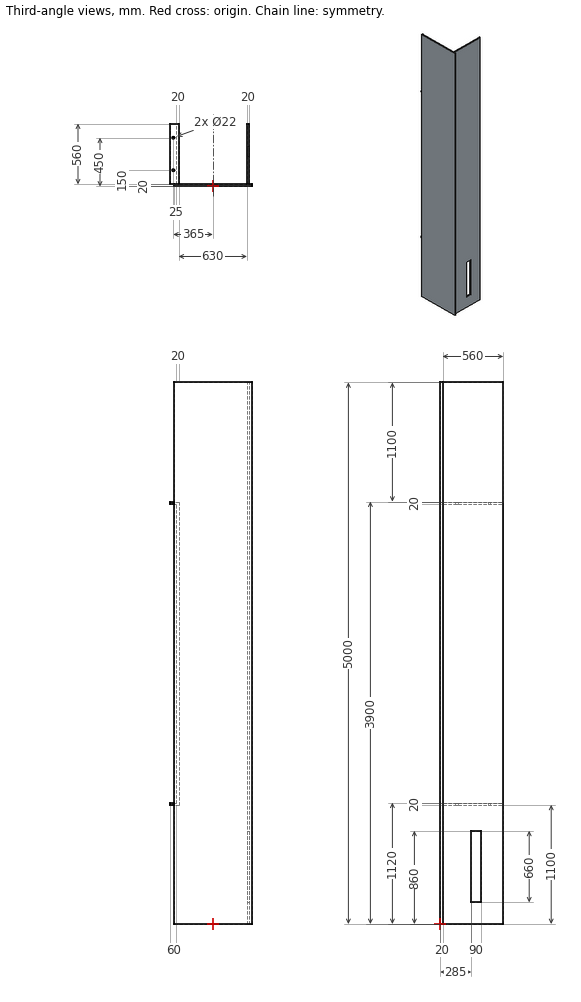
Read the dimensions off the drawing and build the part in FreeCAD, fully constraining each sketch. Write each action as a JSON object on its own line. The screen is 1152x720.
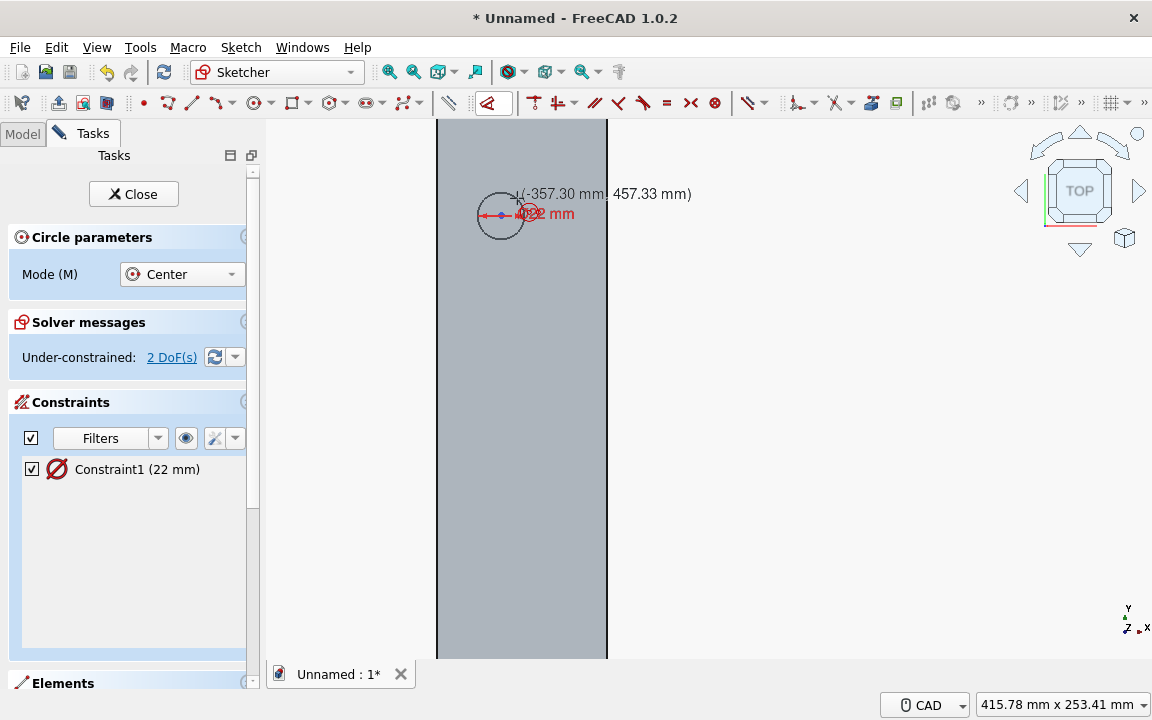
{"action": "scroll", "coordinate": [502, 218], "scroll_direction": "down", "scroll_amount": 5}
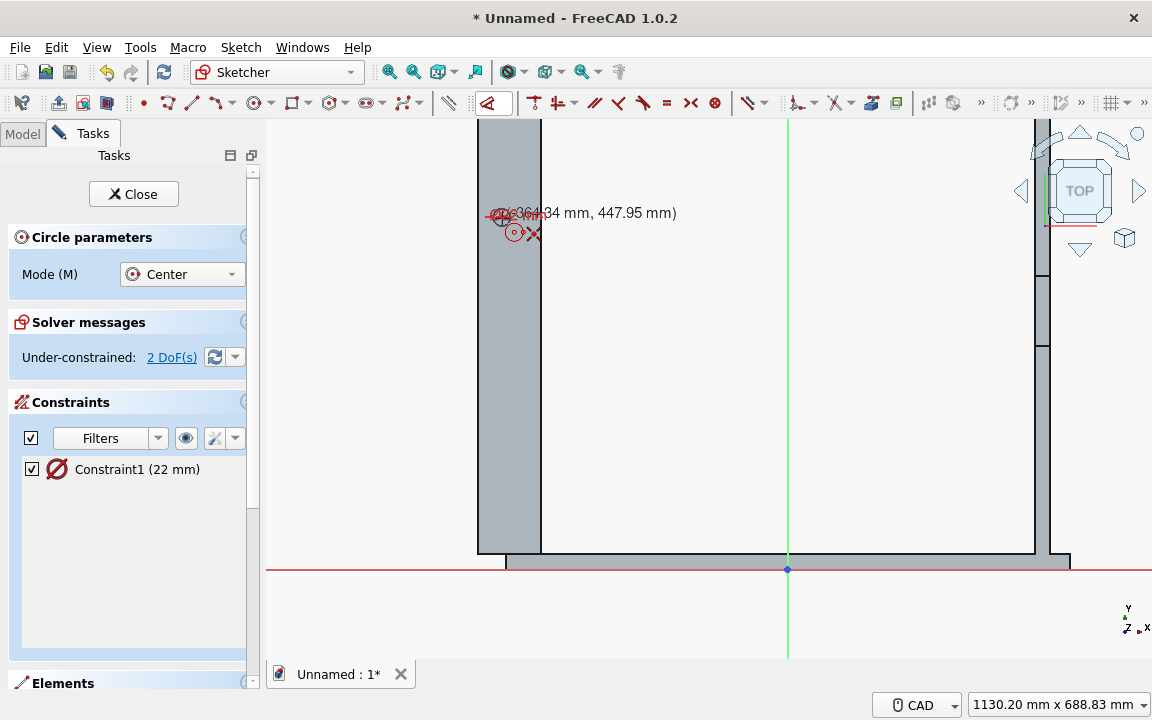
{"action": "scroll", "coordinate": [502, 452], "scroll_direction": "up", "scroll_amount": 5}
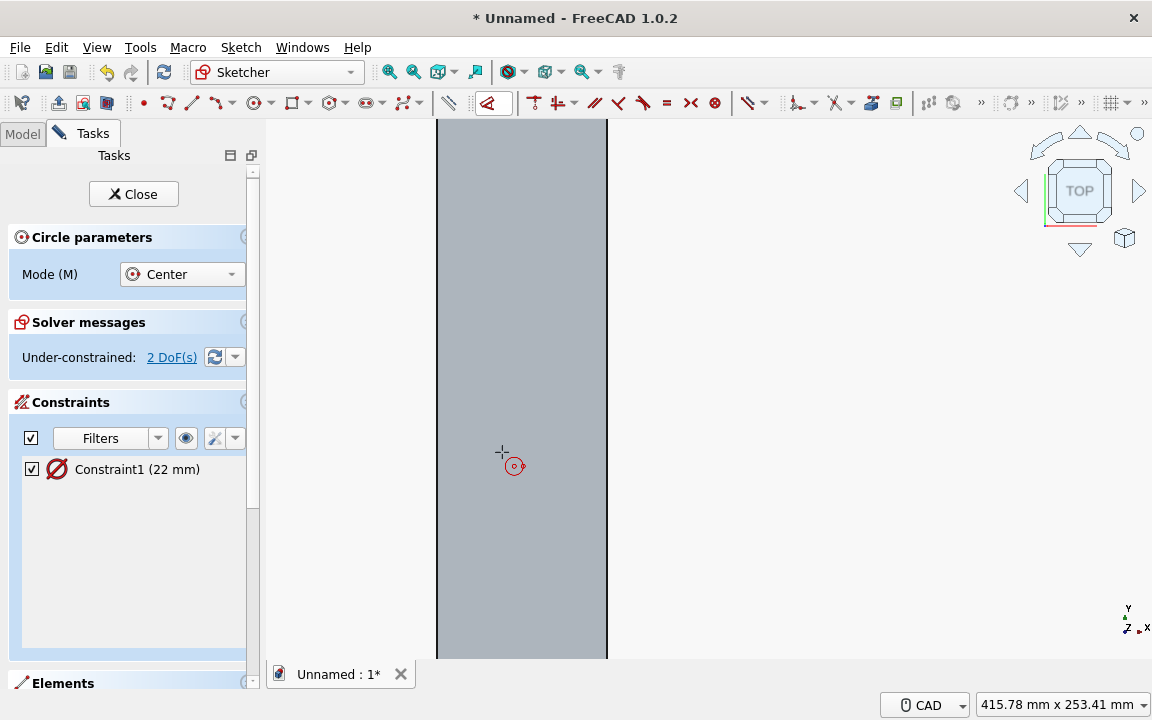
{"action": "left_click", "coordinate": [501, 451]}
{"action": "mouse_move", "coordinate": [517, 435]}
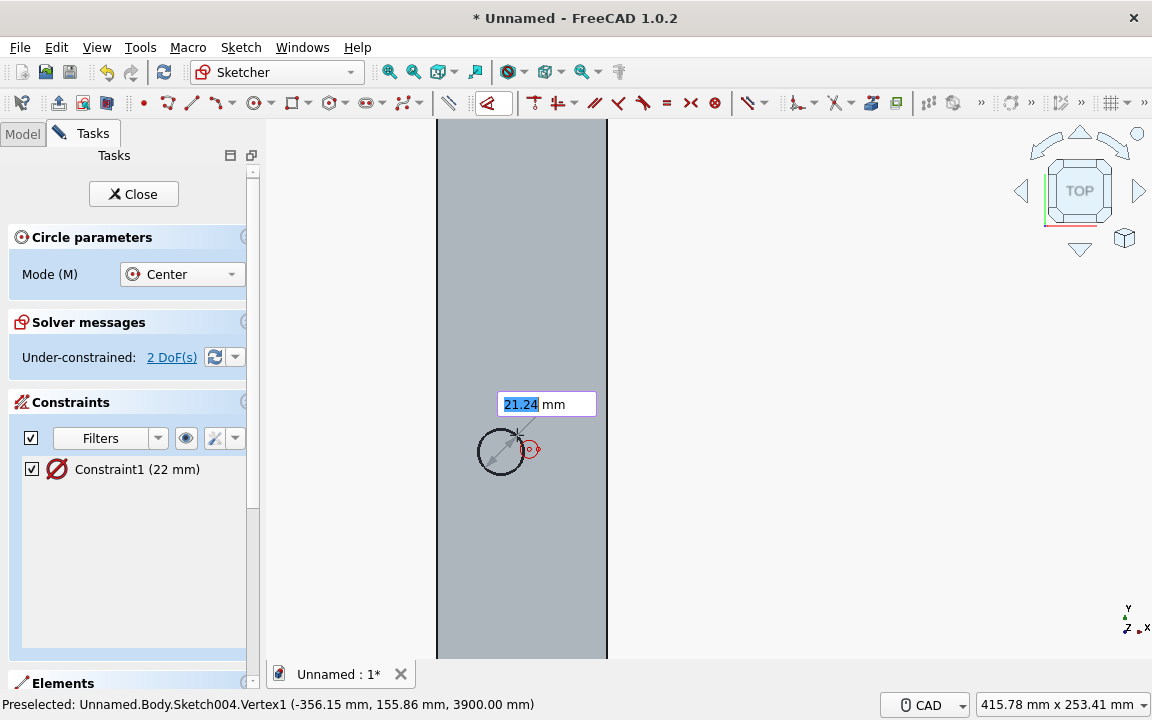
{"action": "type", "text": "22"}
{"action": "key", "text": "Return"}
{"action": "key", "text": "Escape"}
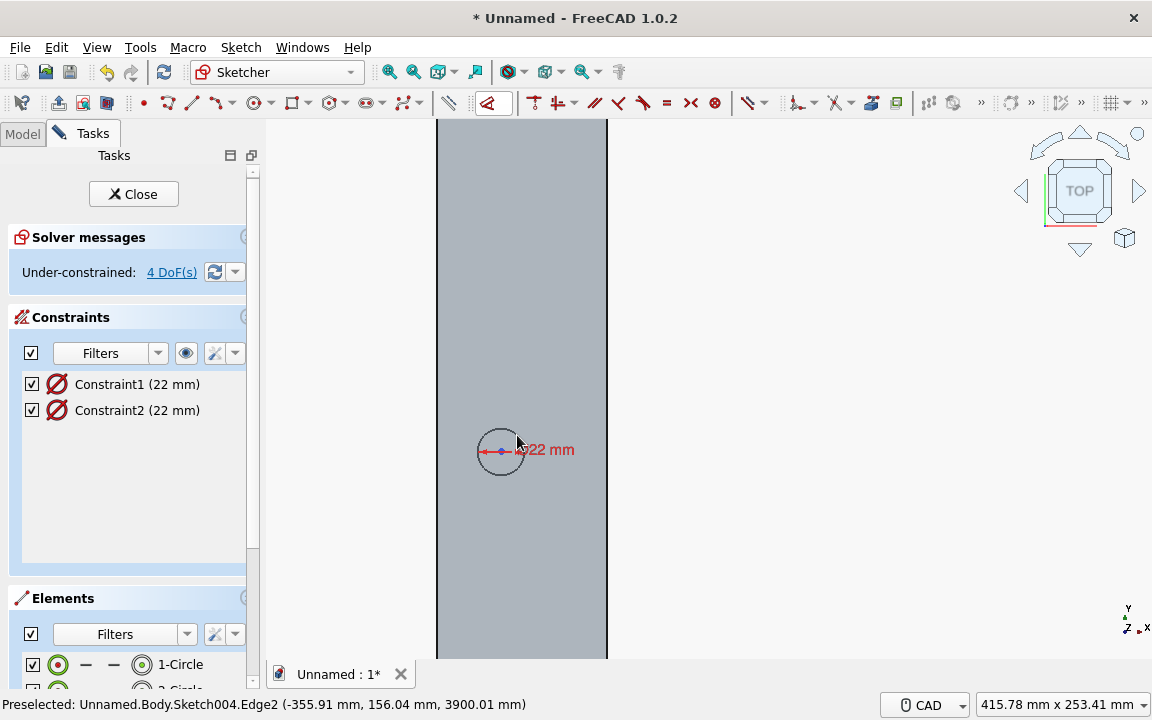
{"action": "scroll", "coordinate": [502, 453], "scroll_direction": "down", "scroll_amount": 5}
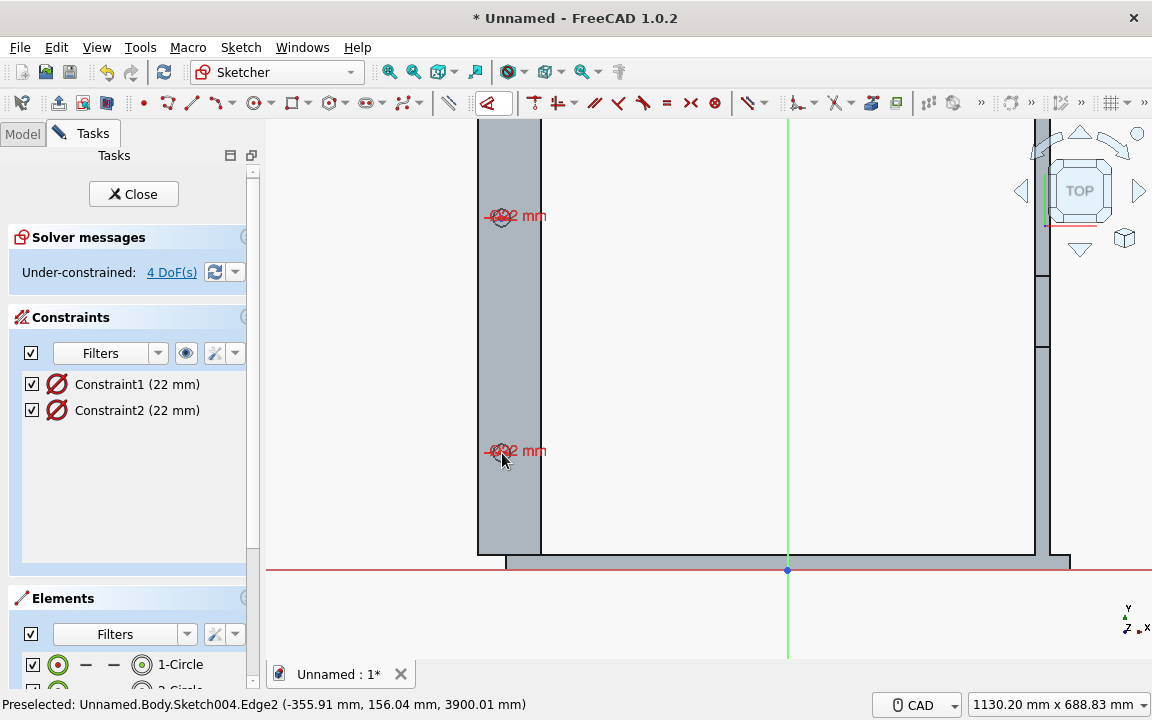
{"action": "left_click", "coordinate": [502, 218]}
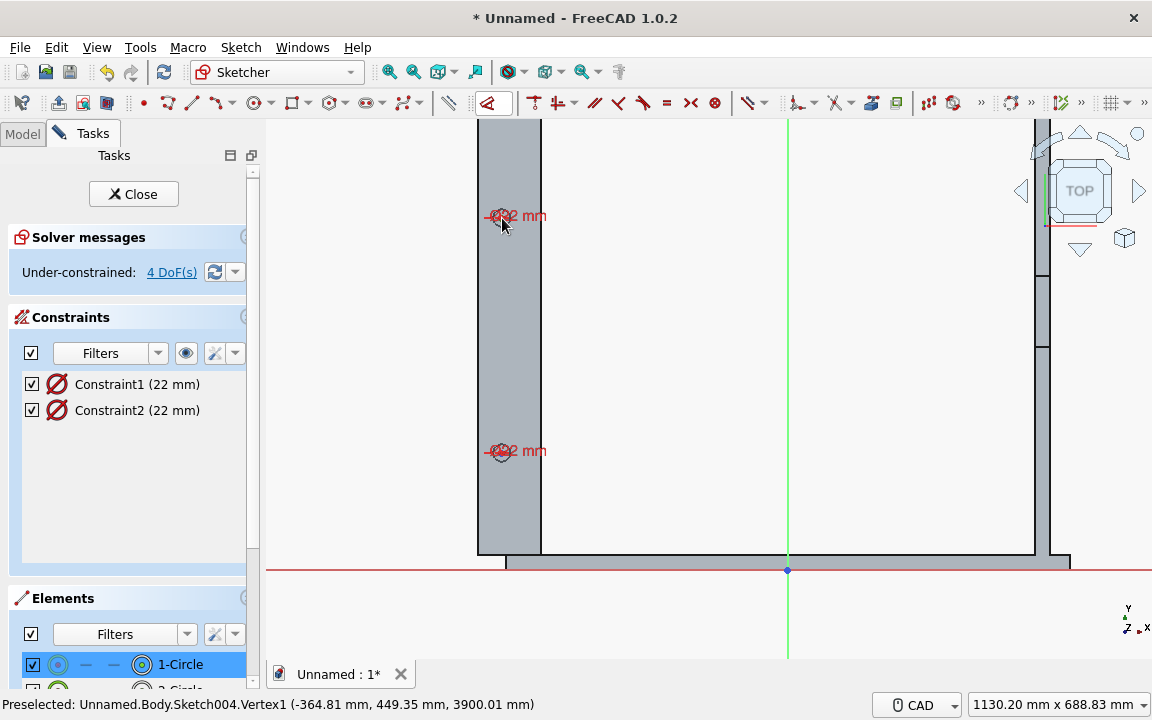
{"action": "key", "text": "l"}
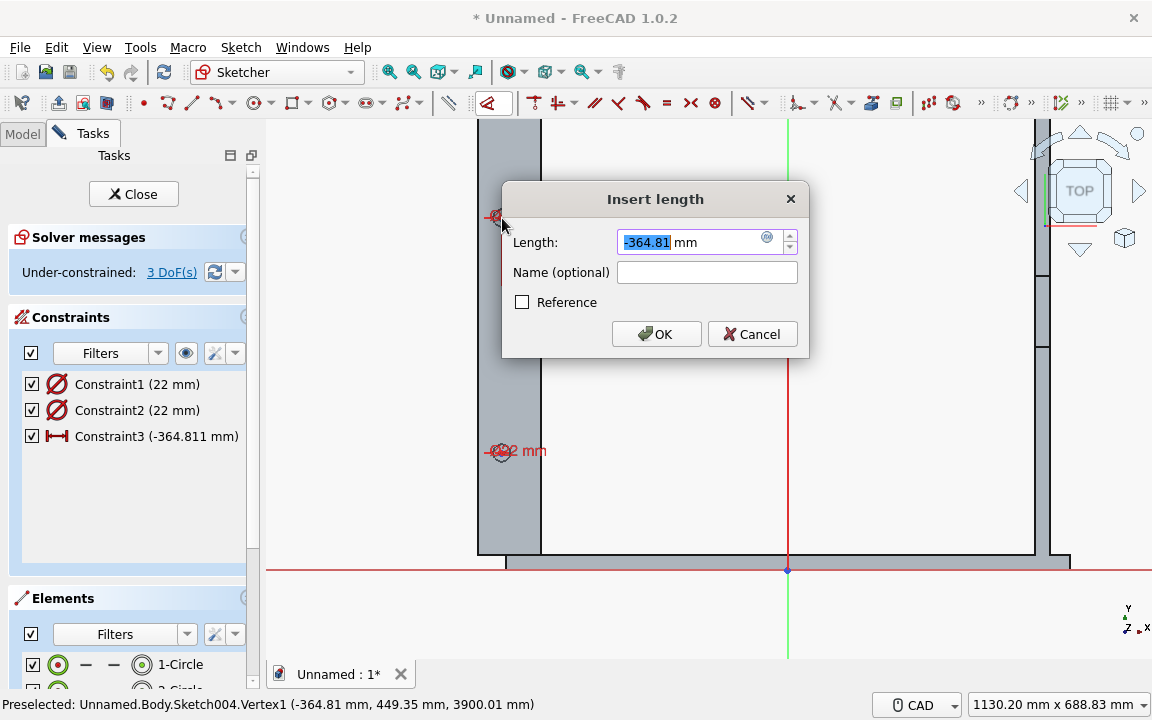
{"action": "type", "text": "-365"}
{"action": "key", "text": "Return"}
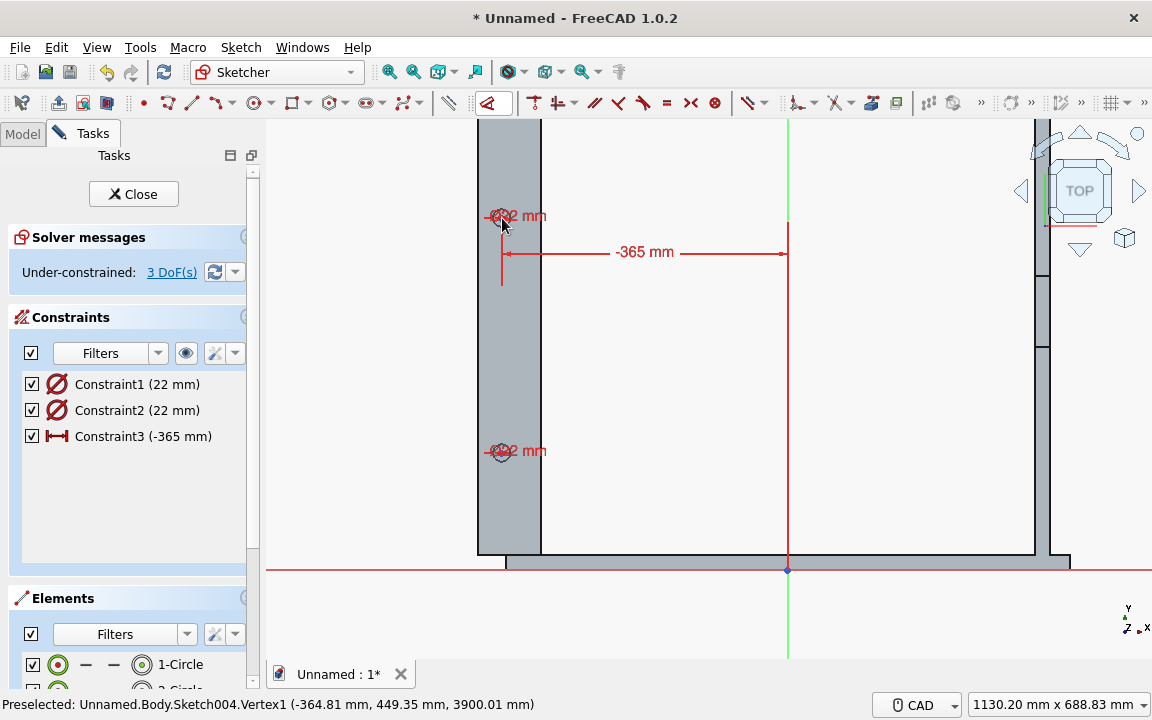
{"action": "left_click", "coordinate": [502, 218]}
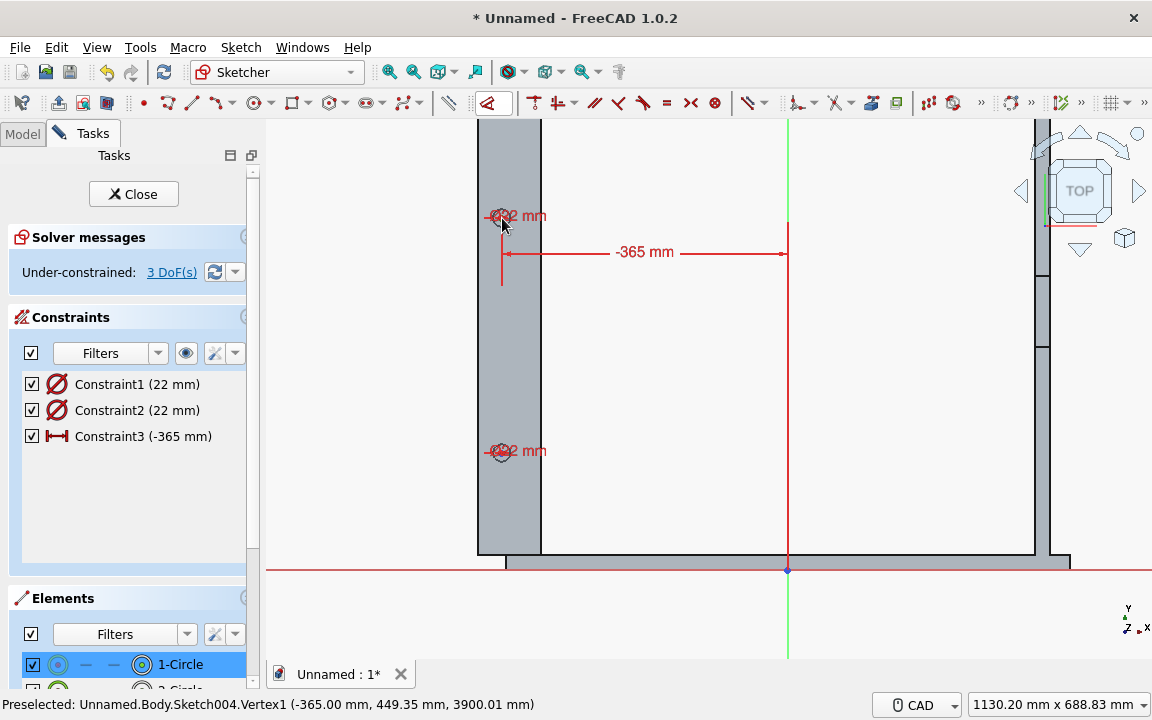
{"action": "left_click", "coordinate": [506, 104]}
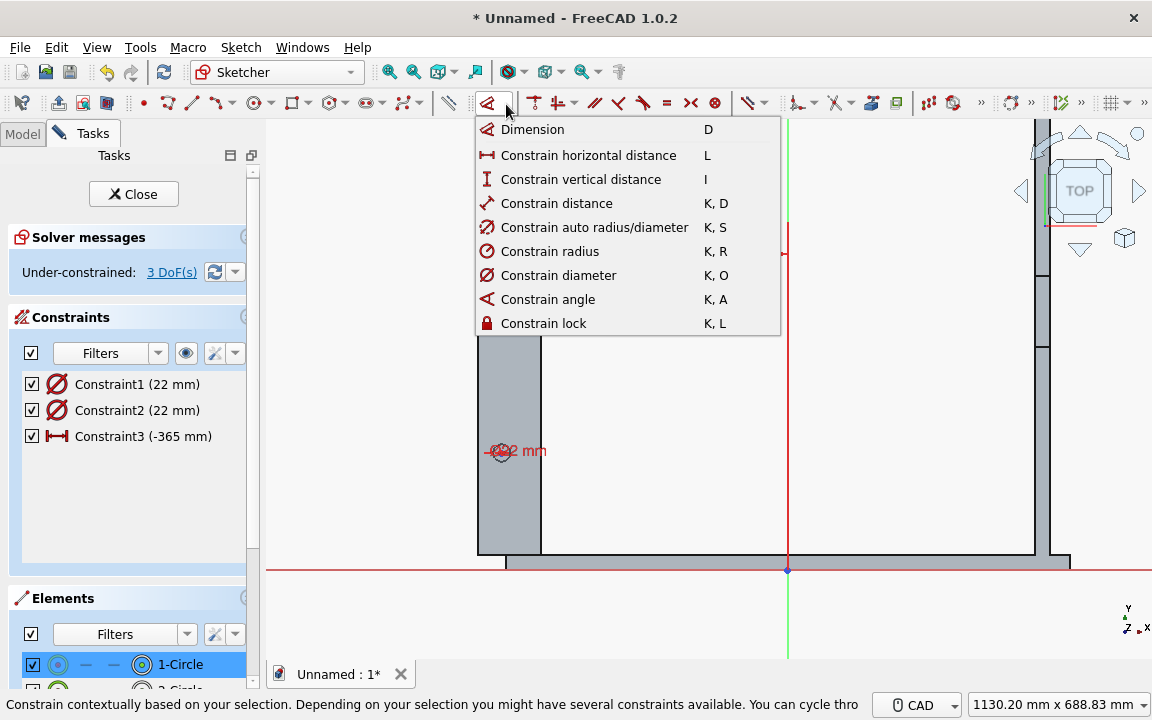
{"action": "left_click", "coordinate": [628, 179]}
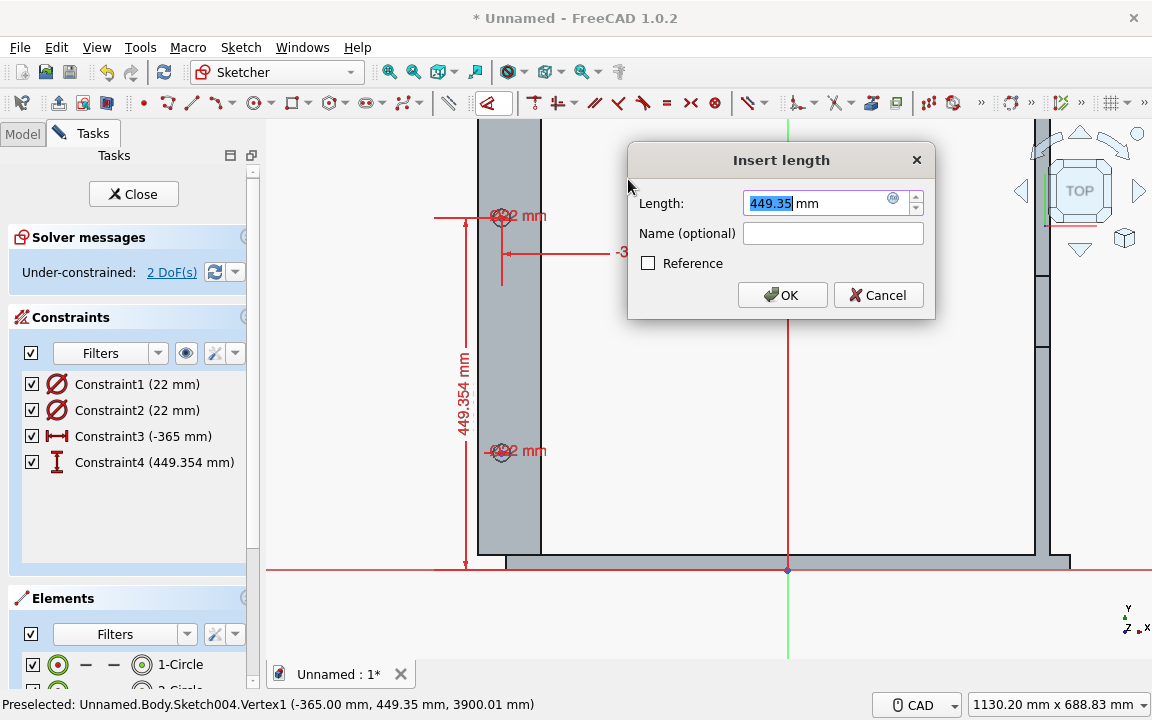
{"action": "type", "text": "450"}
{"action": "key", "text": "Return"}